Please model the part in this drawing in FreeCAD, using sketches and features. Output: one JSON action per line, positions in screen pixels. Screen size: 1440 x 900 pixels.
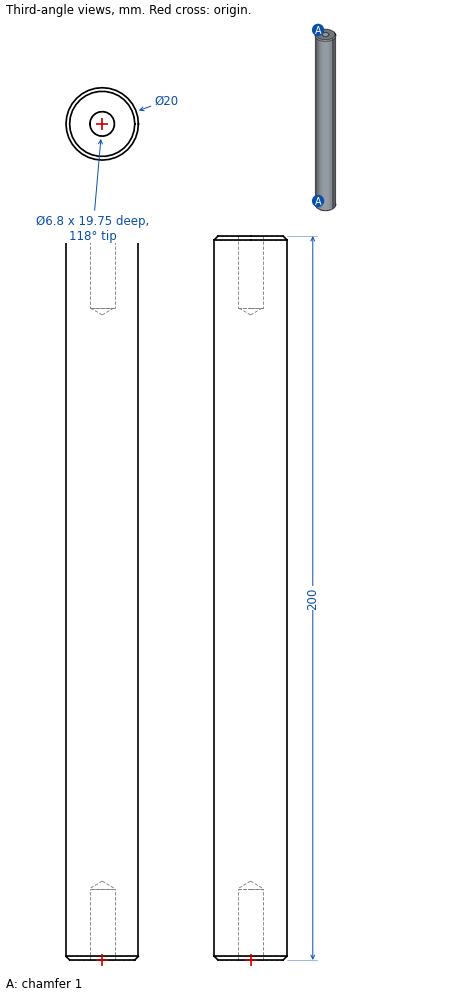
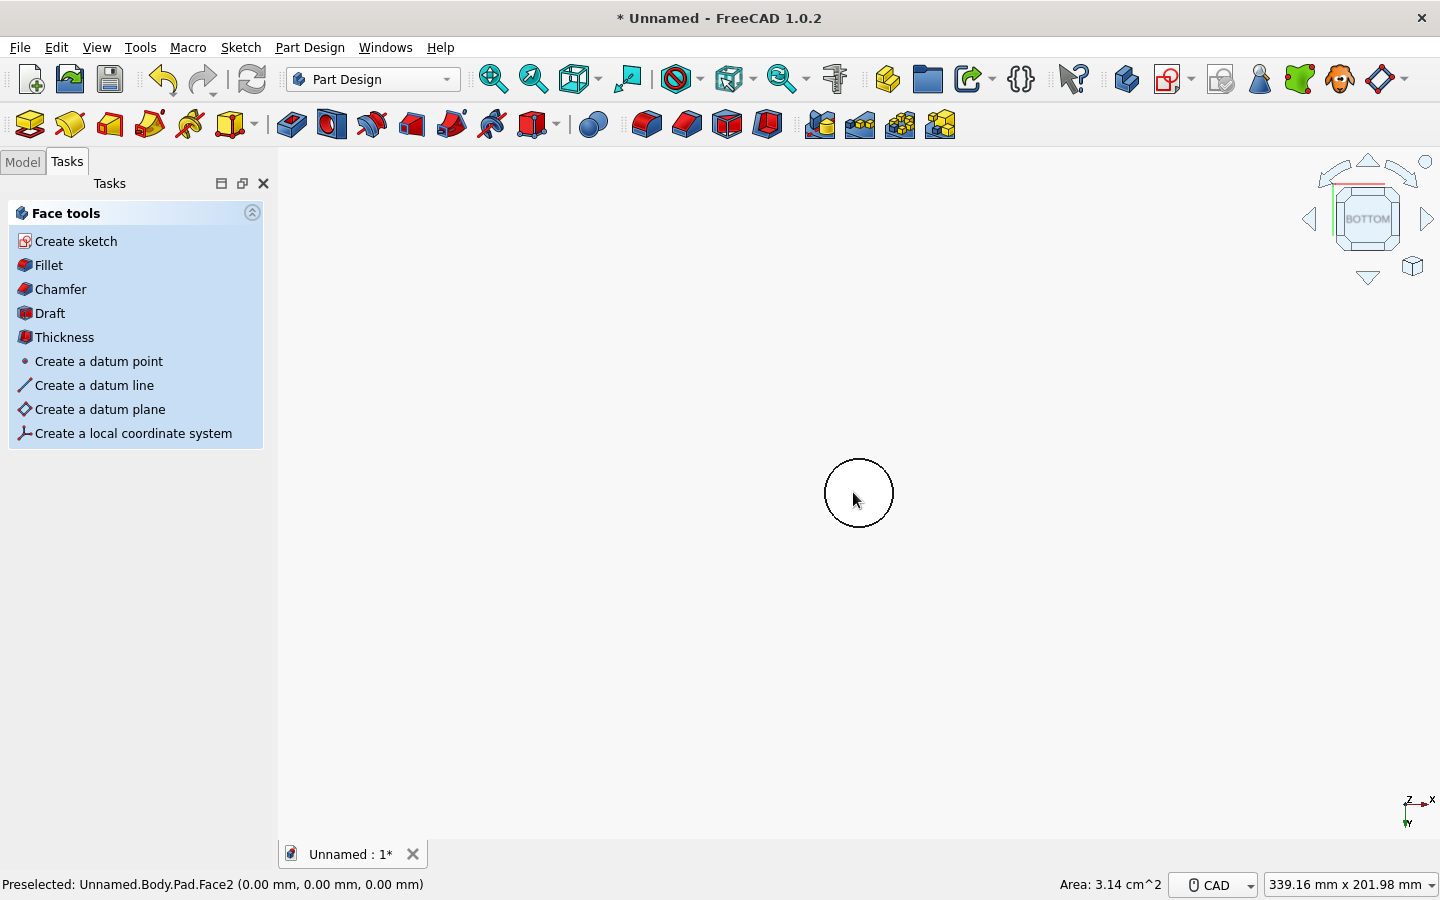
{"action": "left_click", "coordinate": [1168, 80]}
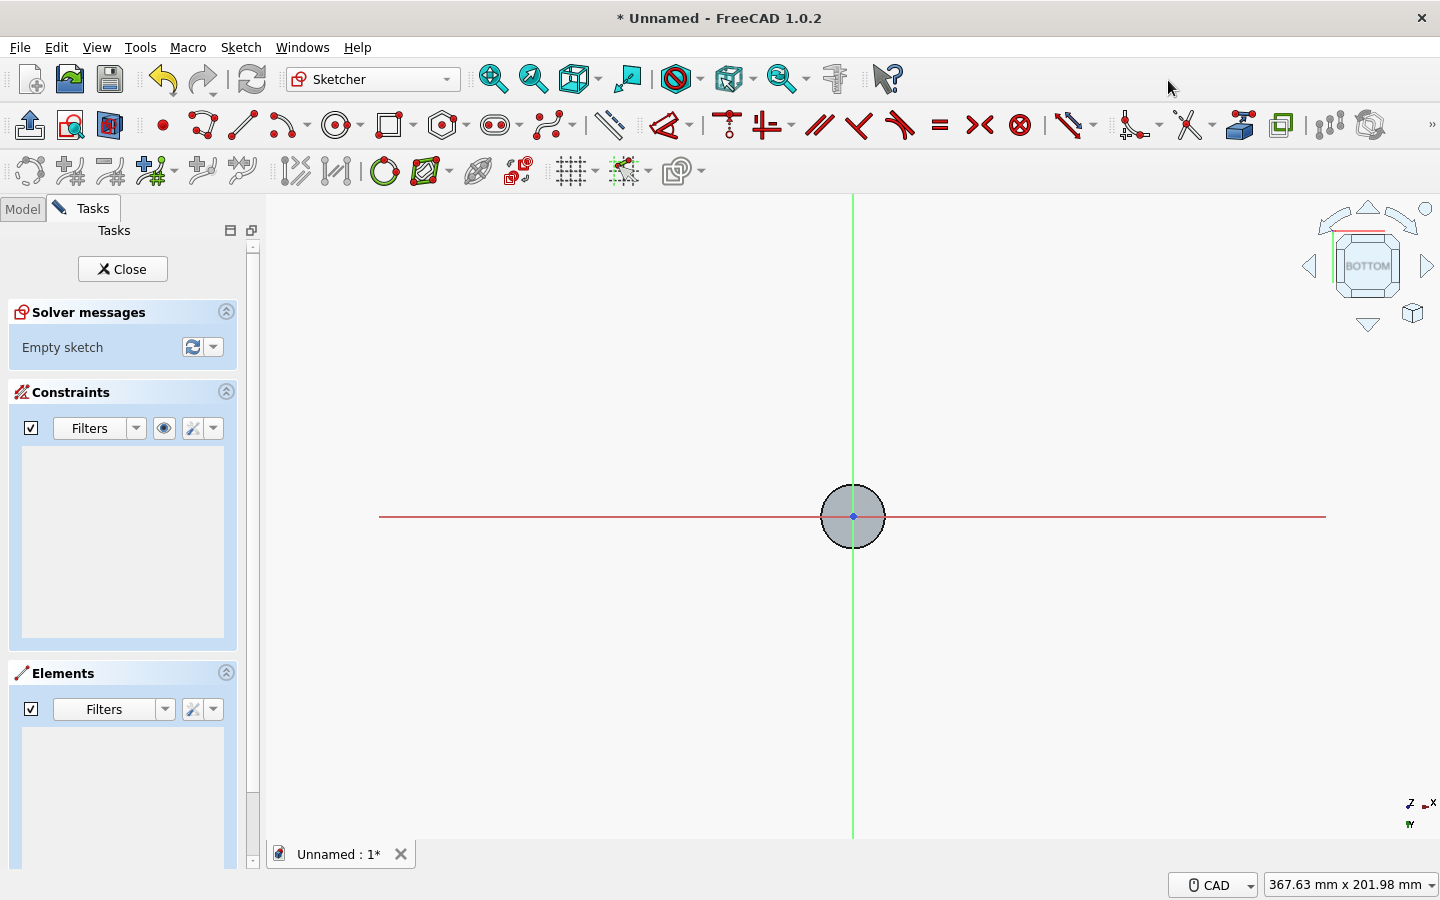
{"action": "scroll", "coordinate": [857, 516], "scroll_direction": "up", "scroll_amount": 15}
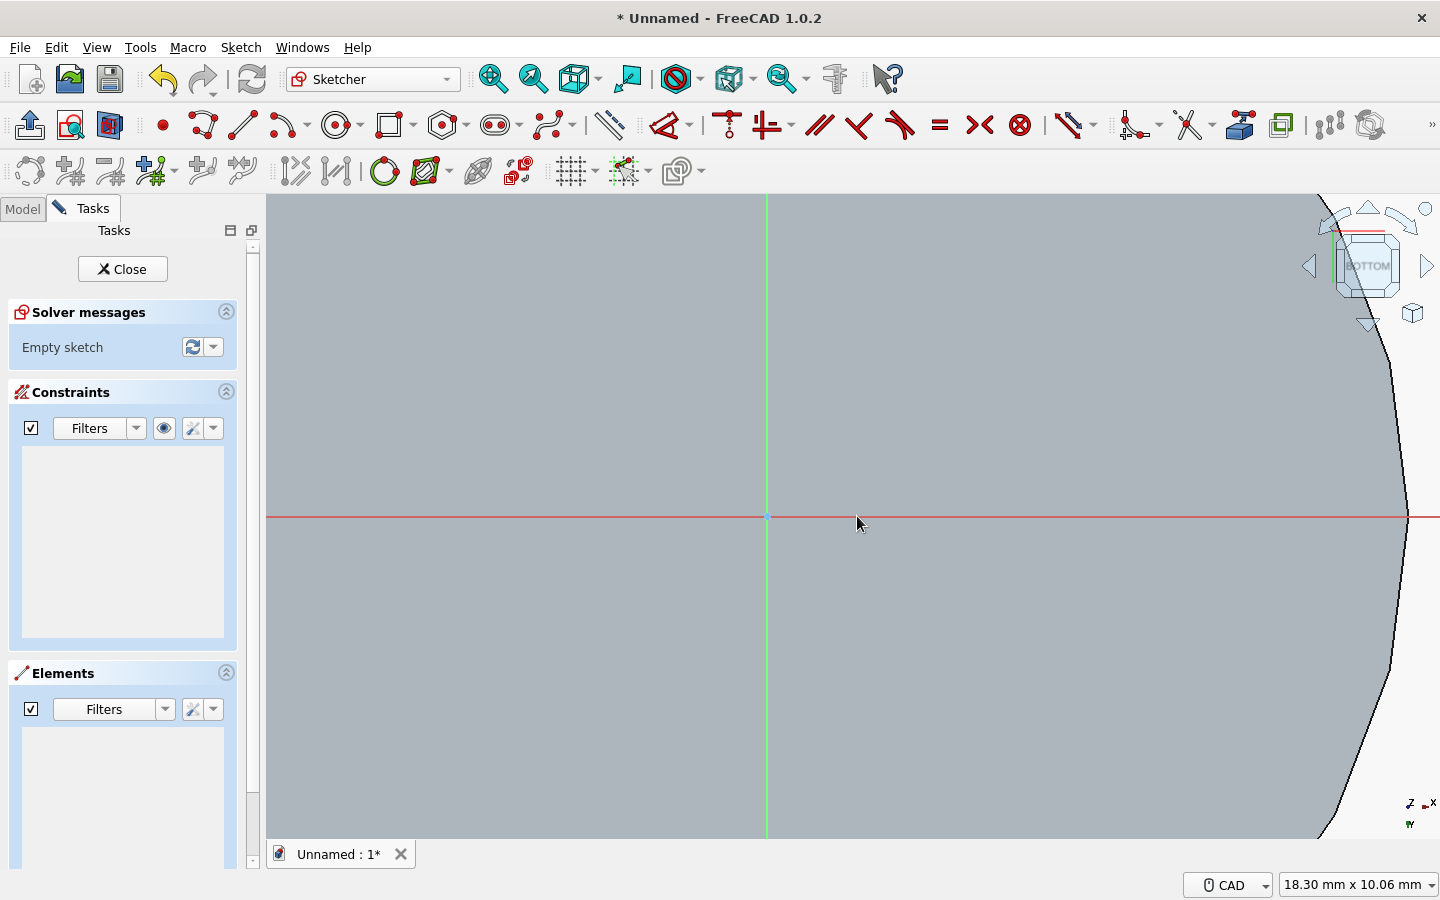
{"action": "key", "text": "g c"}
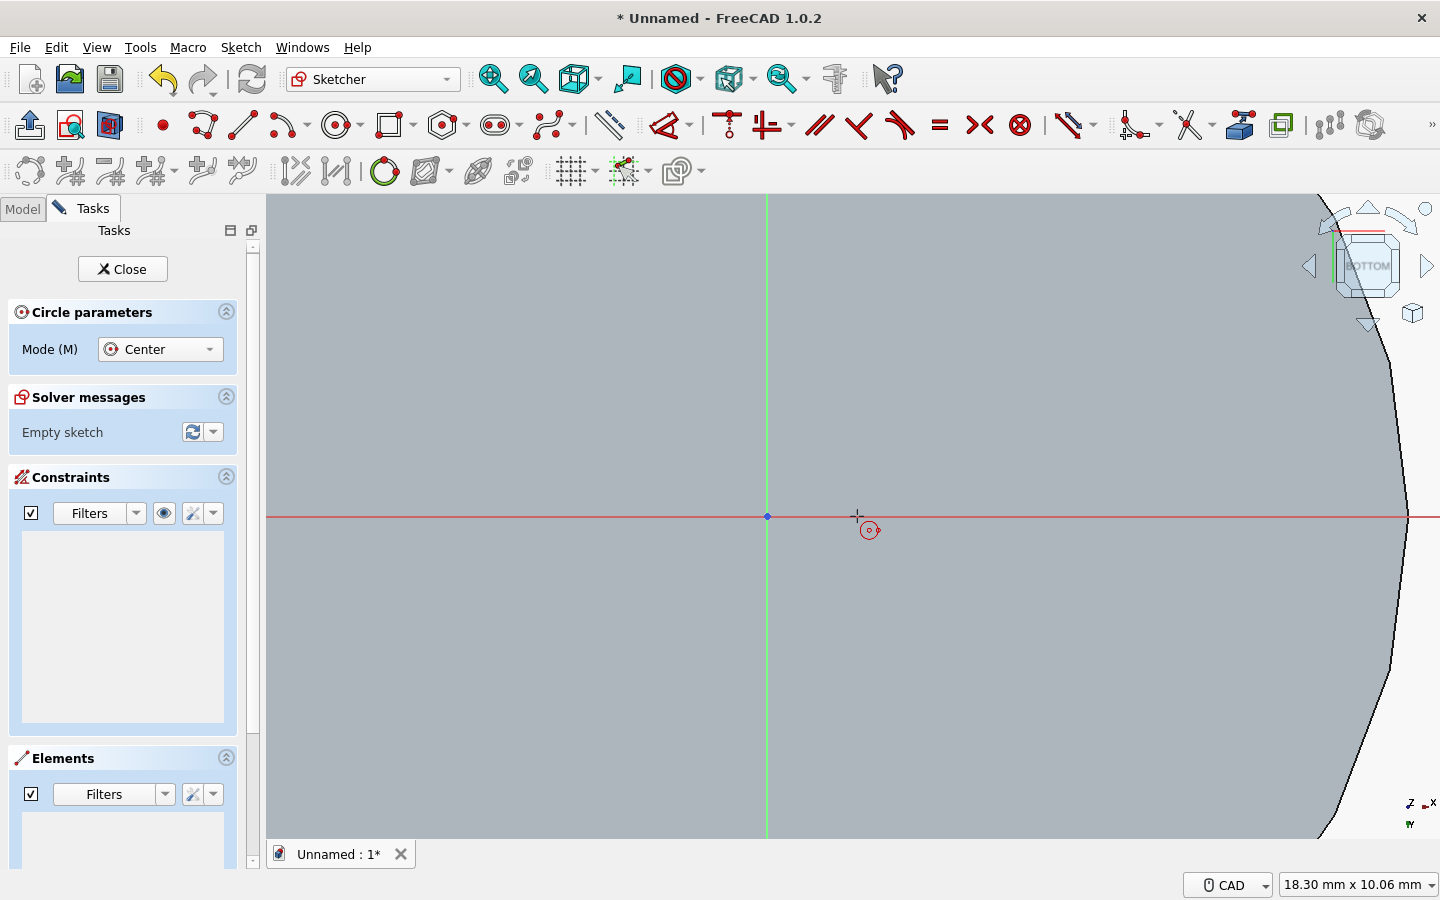
{"action": "left_click", "coordinate": [767, 516]}
{"action": "mouse_move", "coordinate": [921, 362]}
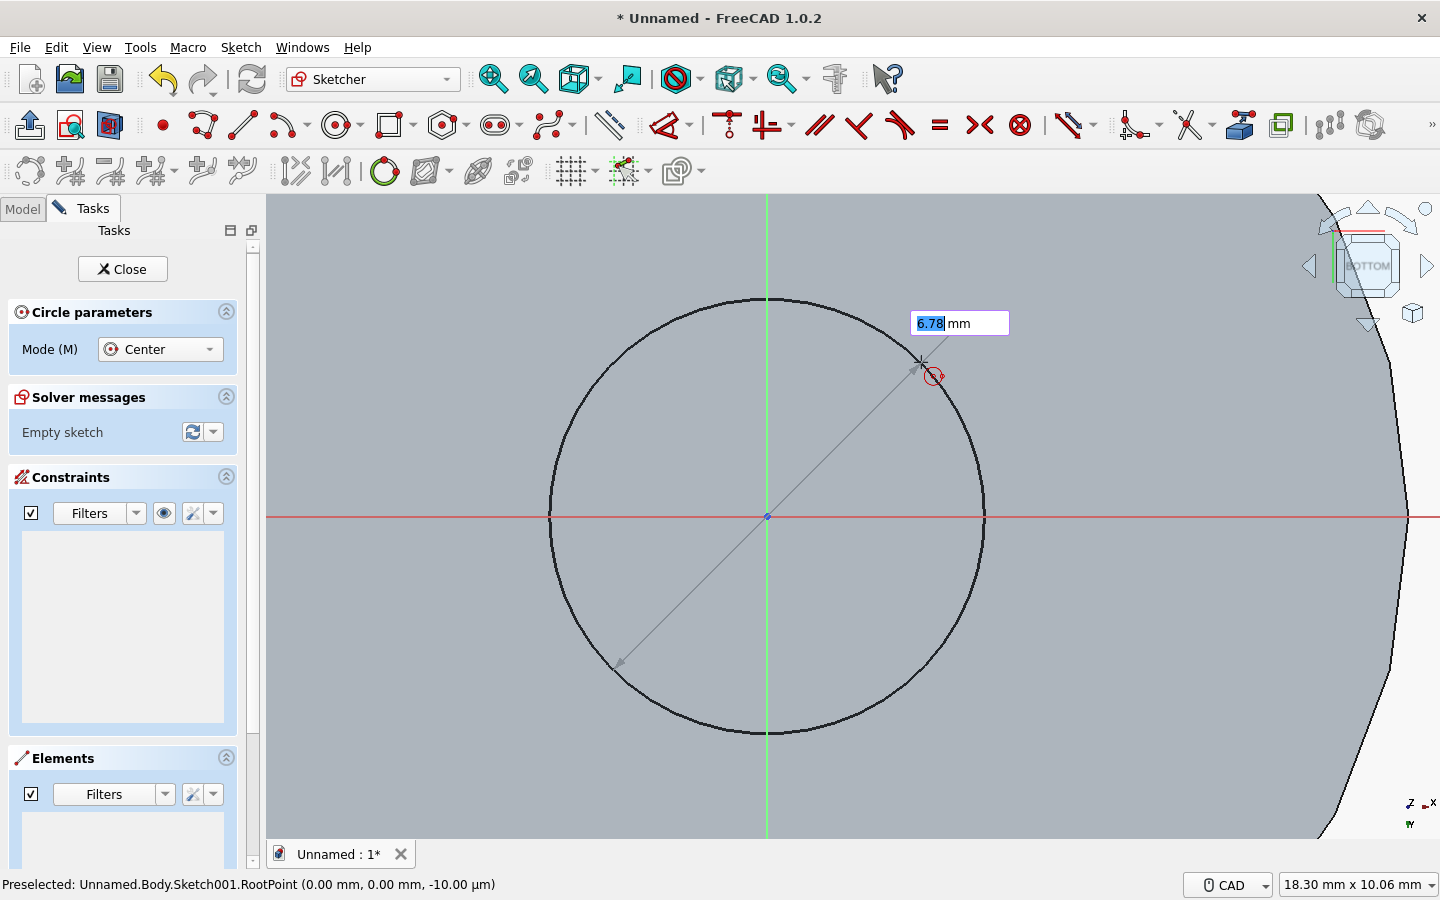
{"action": "type", "text": "6.8"}
{"action": "key", "text": "Return"}
{"action": "key", "text": "Escape"}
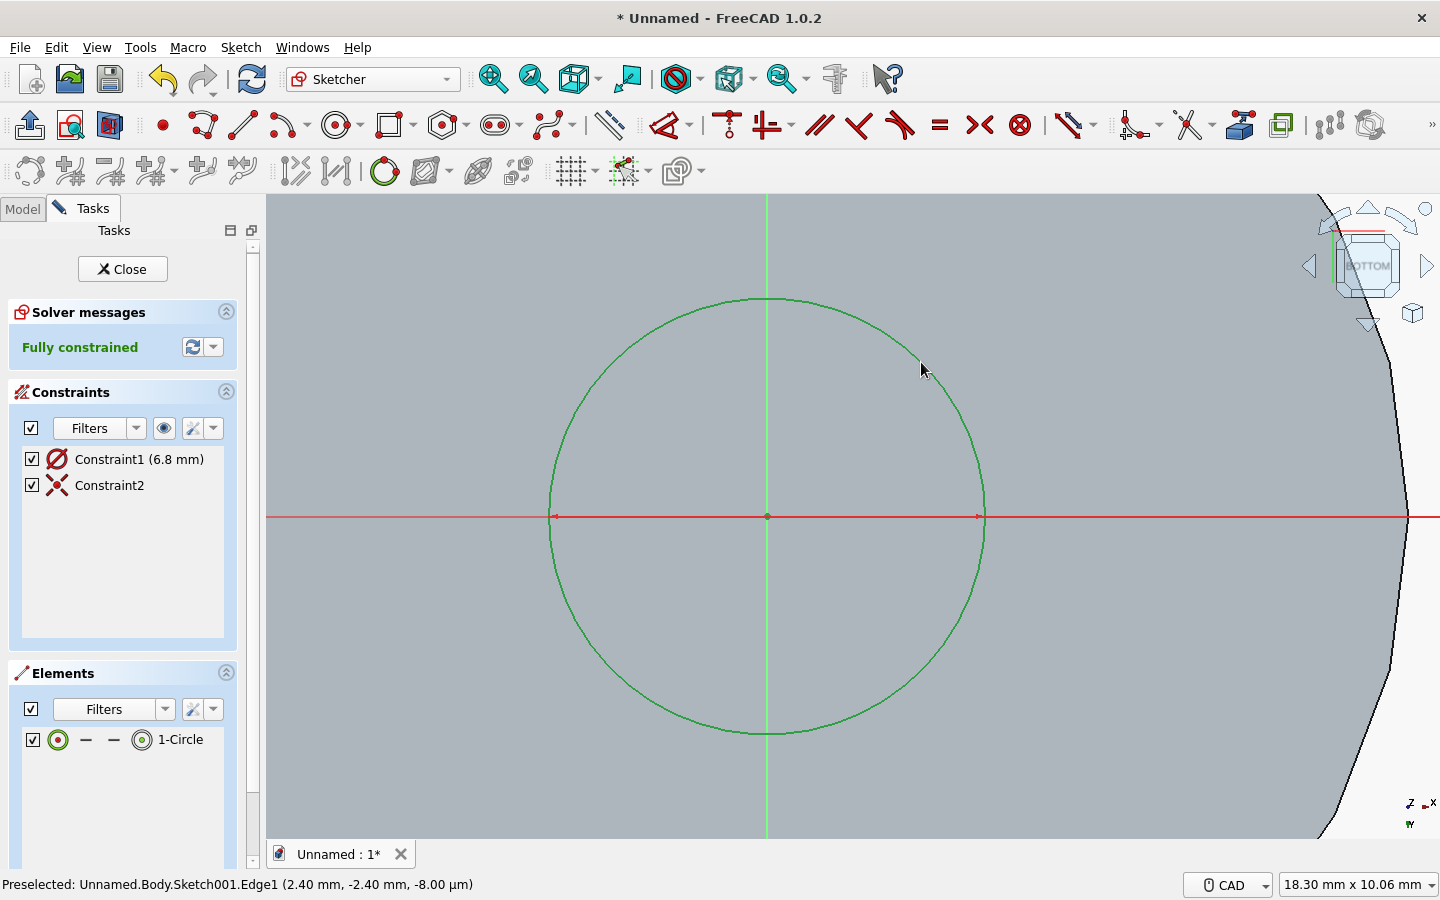
{"action": "left_click", "coordinate": [123, 269]}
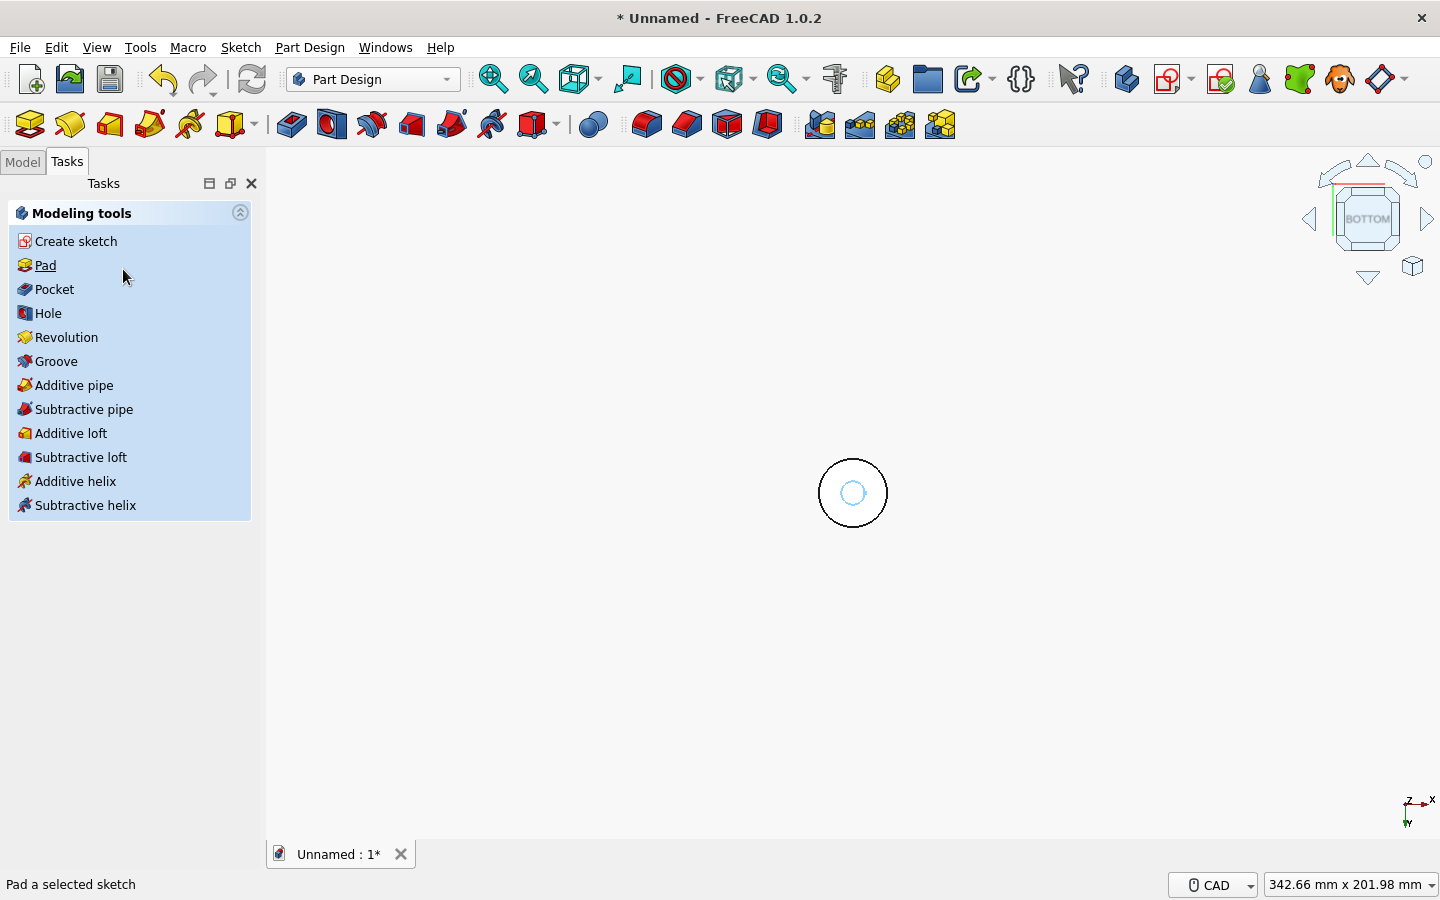
{"action": "left_click", "coordinate": [332, 124]}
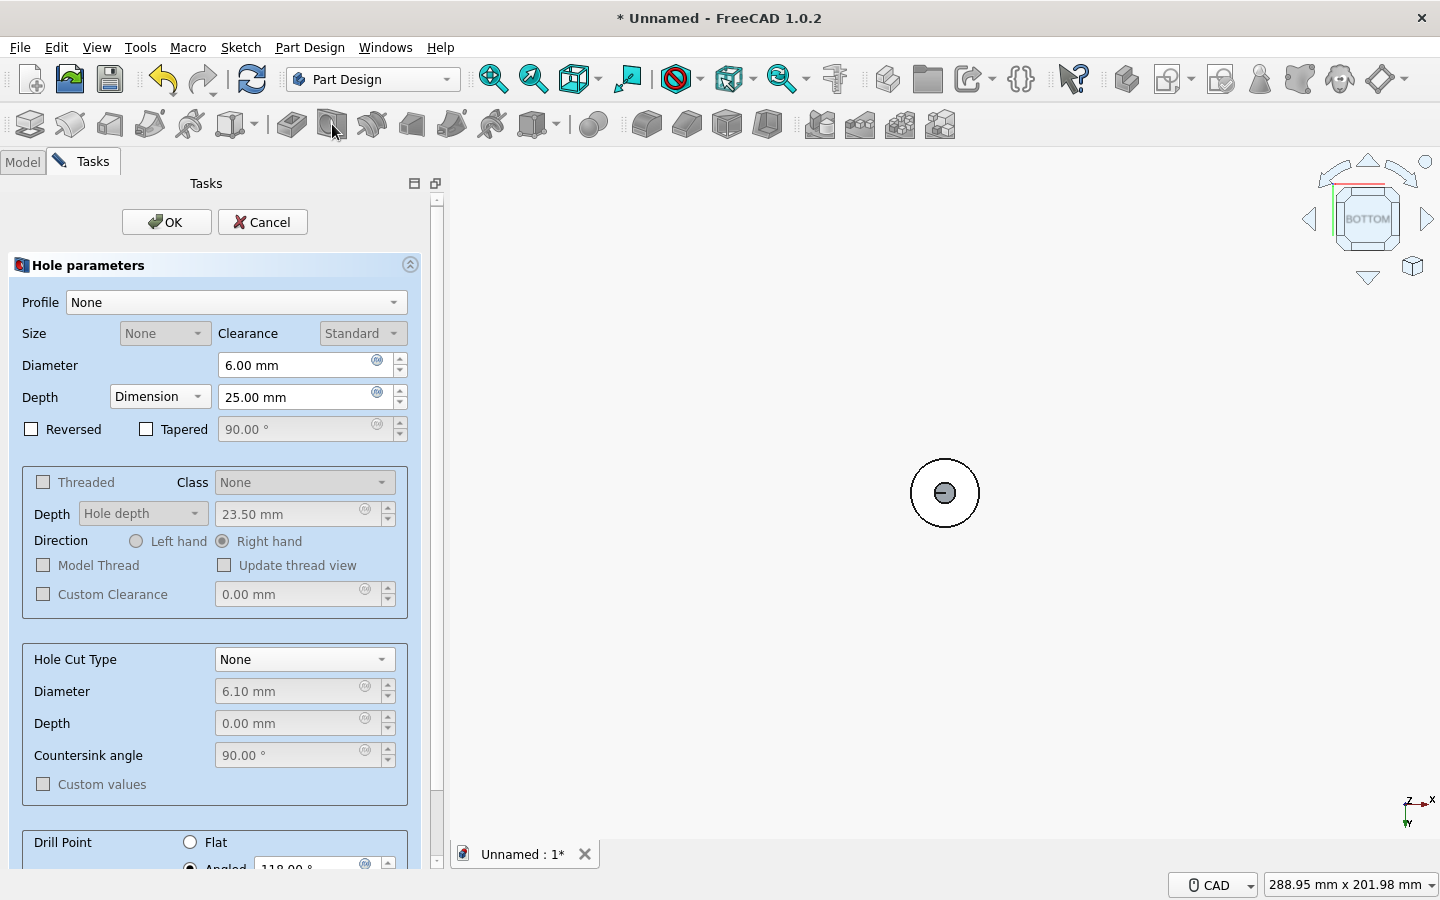
{"action": "triple_click", "coordinate": [305, 365]}